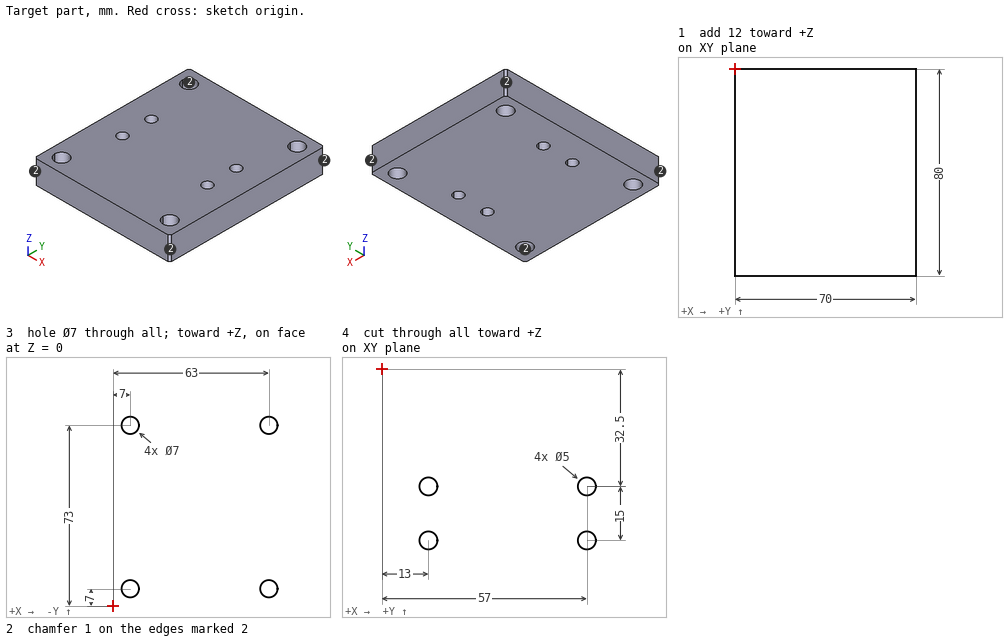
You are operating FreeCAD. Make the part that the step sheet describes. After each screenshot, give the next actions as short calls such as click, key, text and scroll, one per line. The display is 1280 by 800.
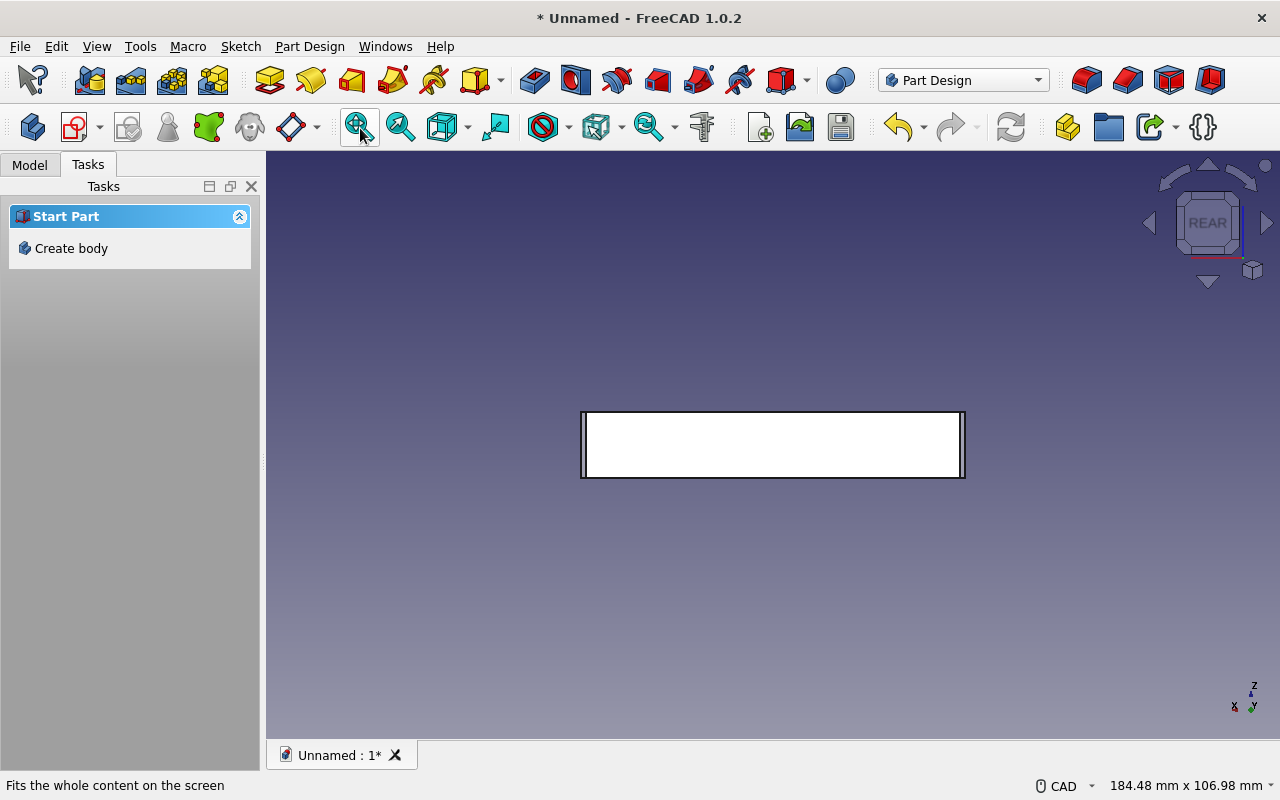
key(5)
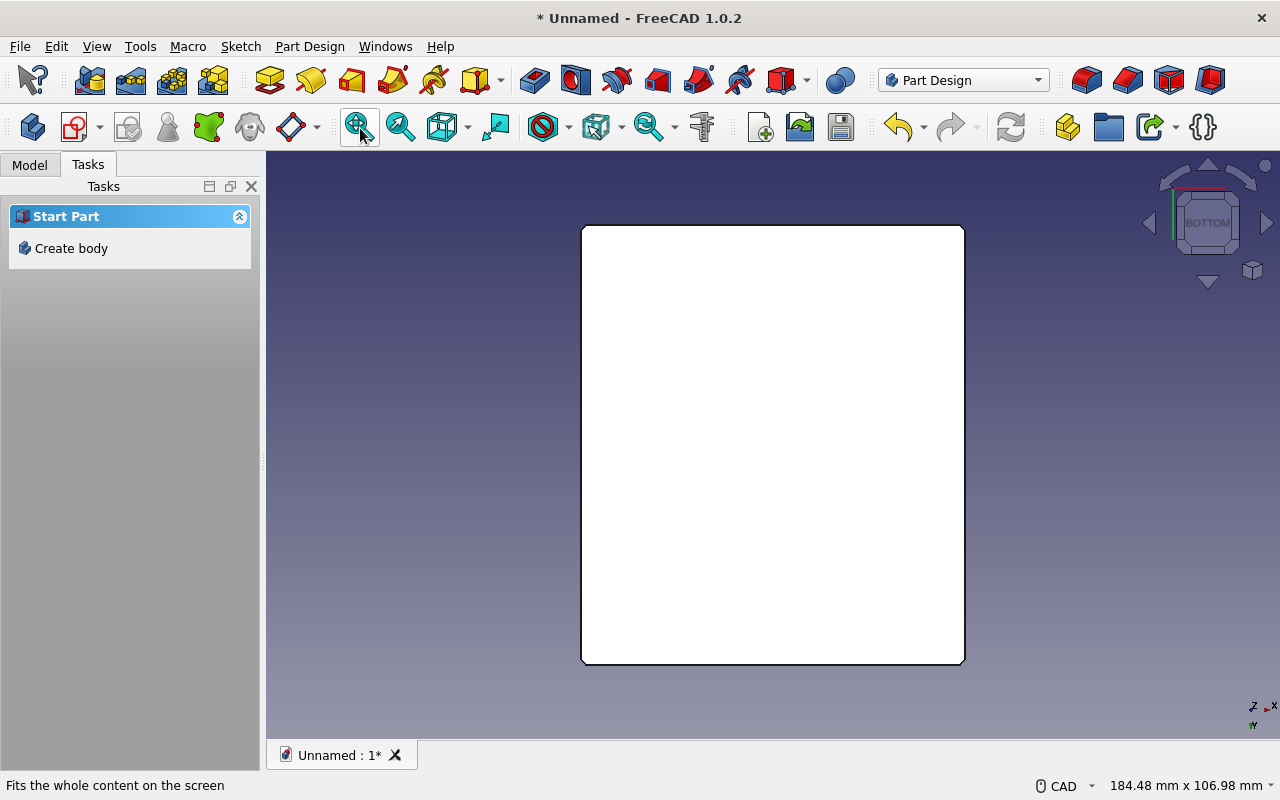
click(773, 444)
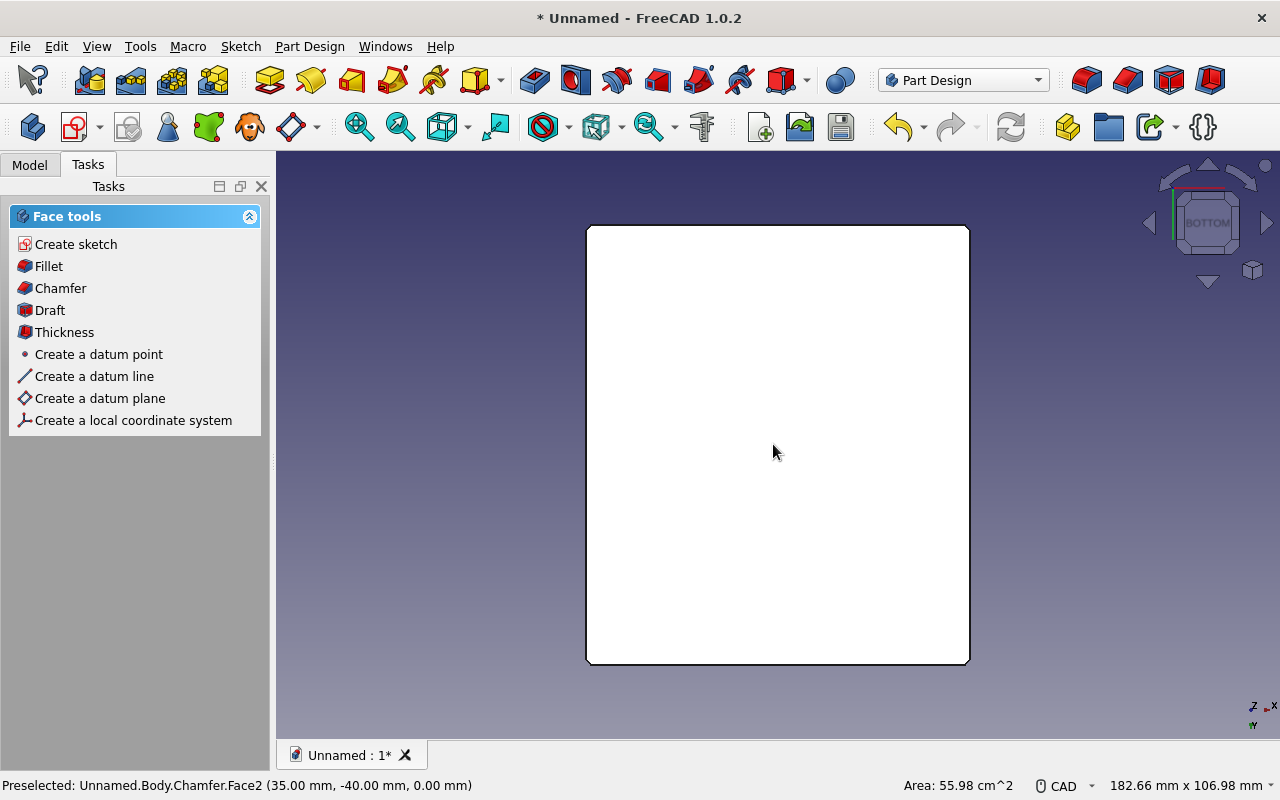
click(74, 128)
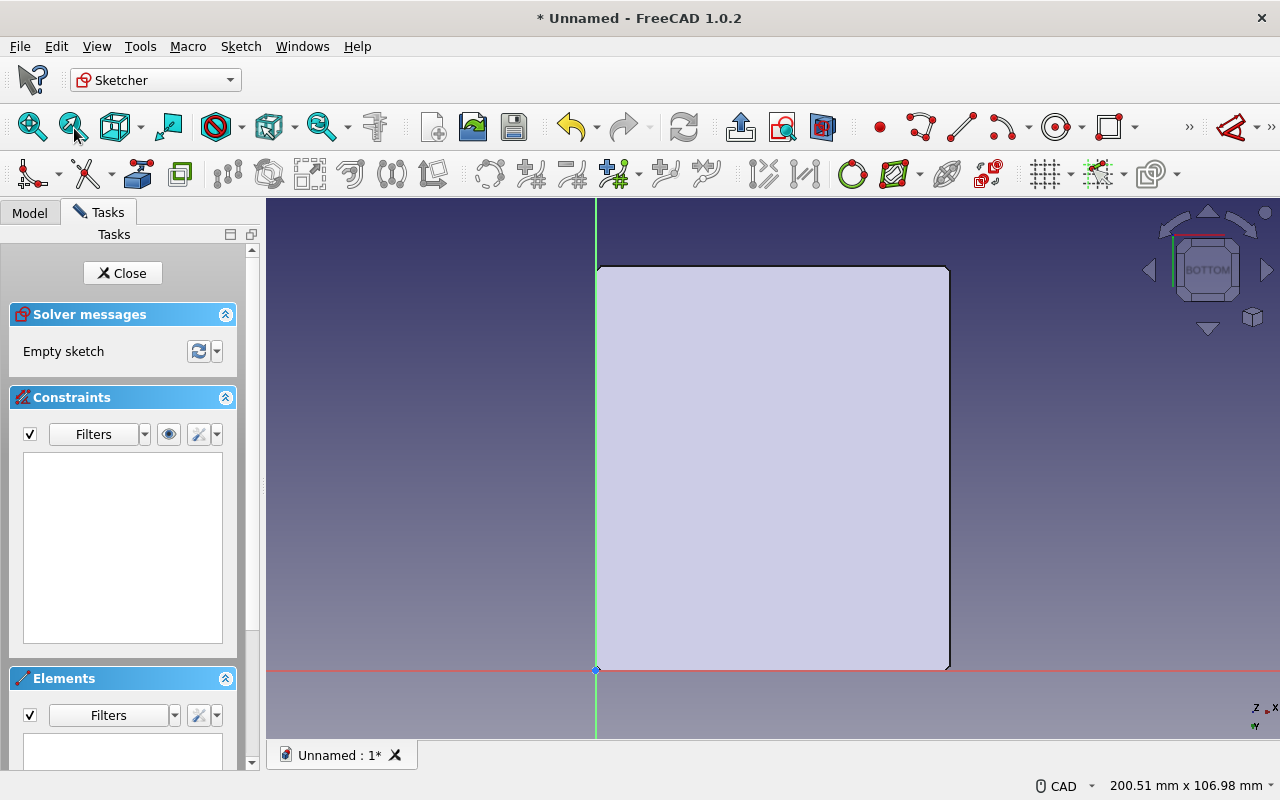
click(1056, 128)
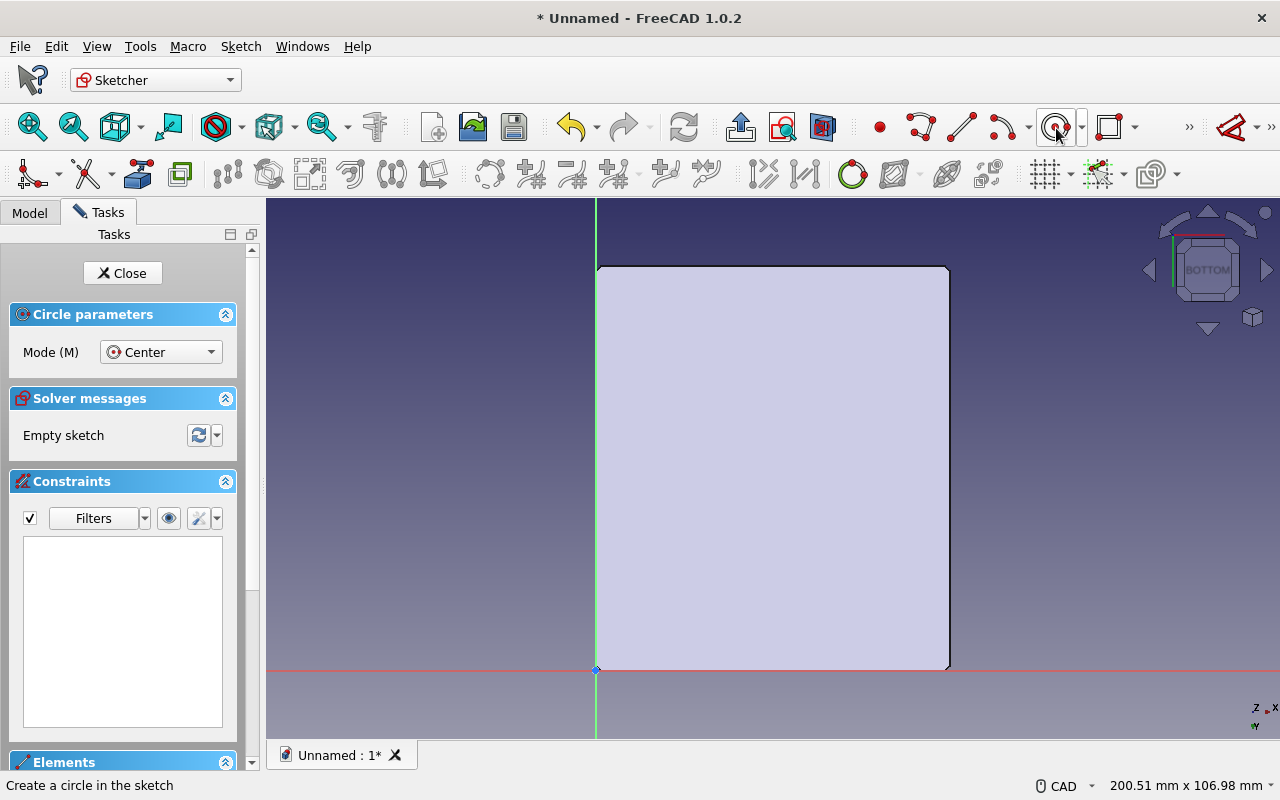
scroll(631, 302, up, 2)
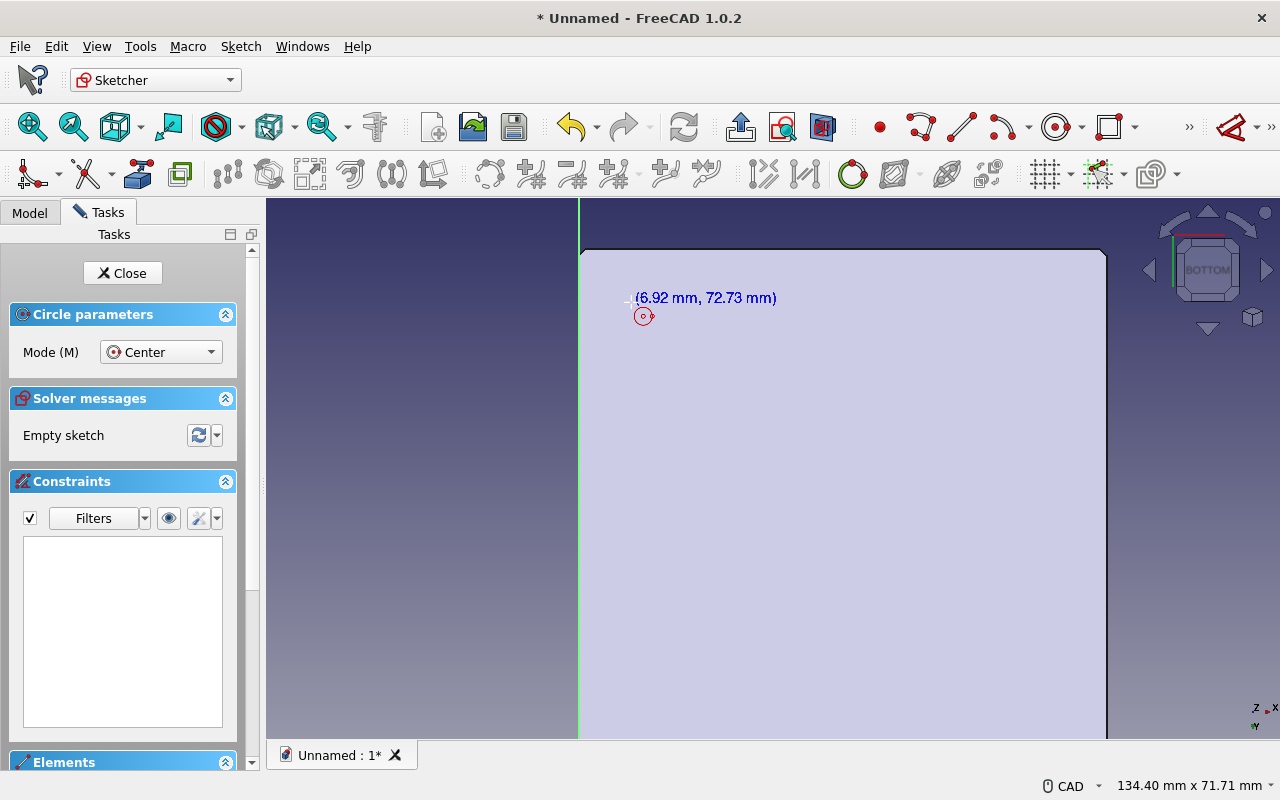
click(631, 301)
move(650, 283)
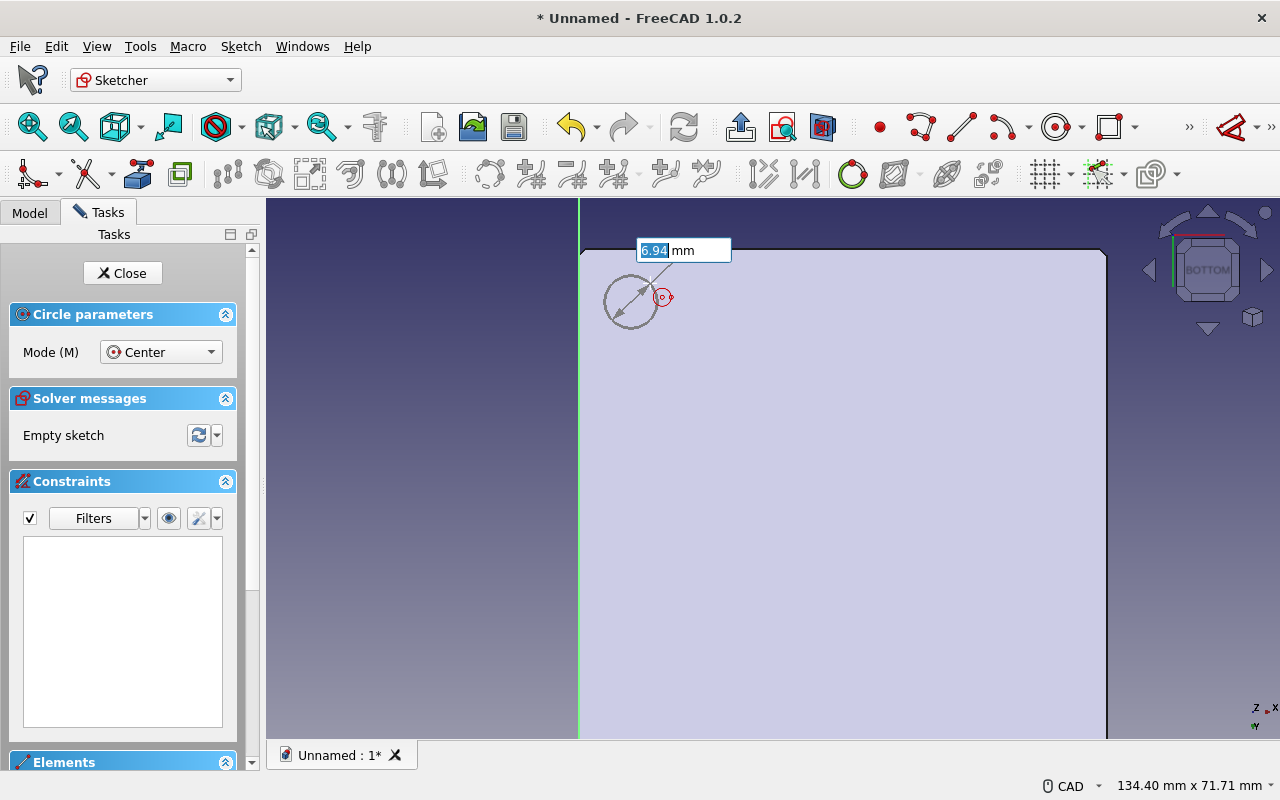
text(7)
key(Return)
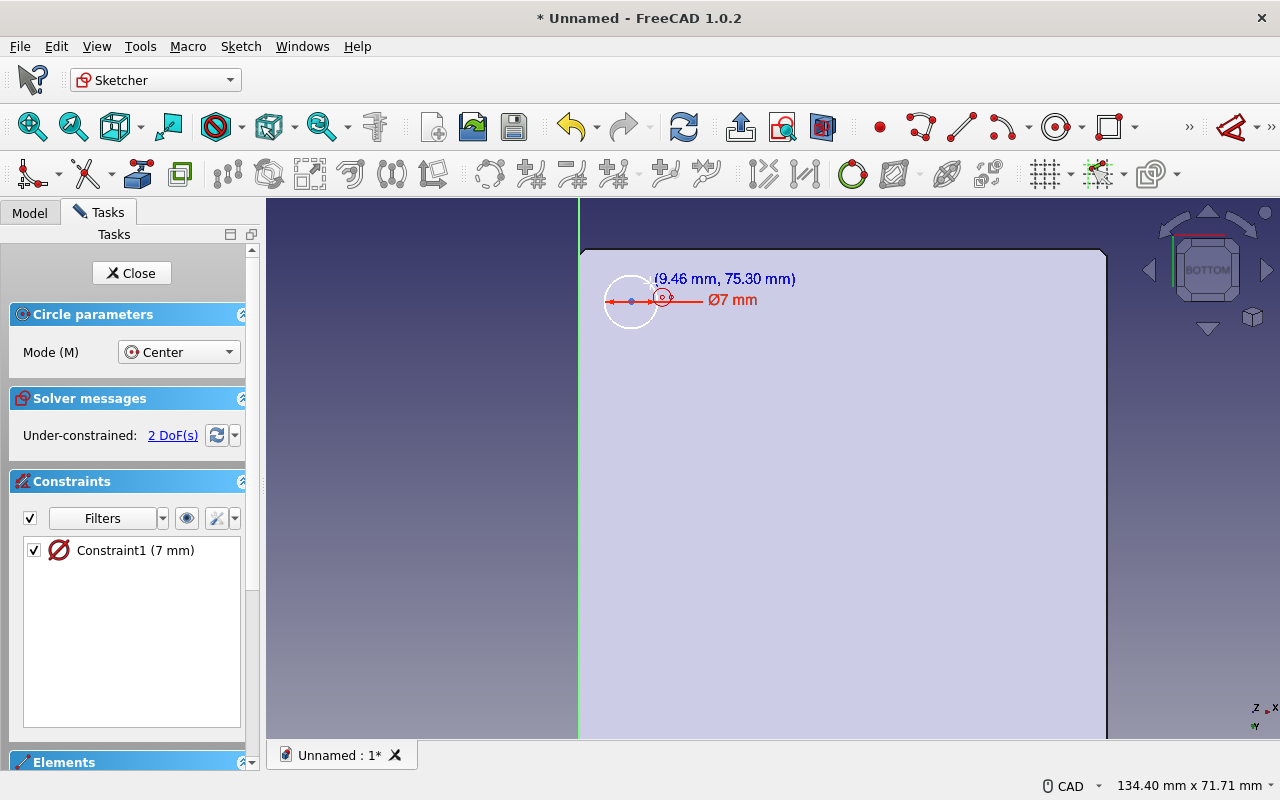
scroll(553, 353, down, 3)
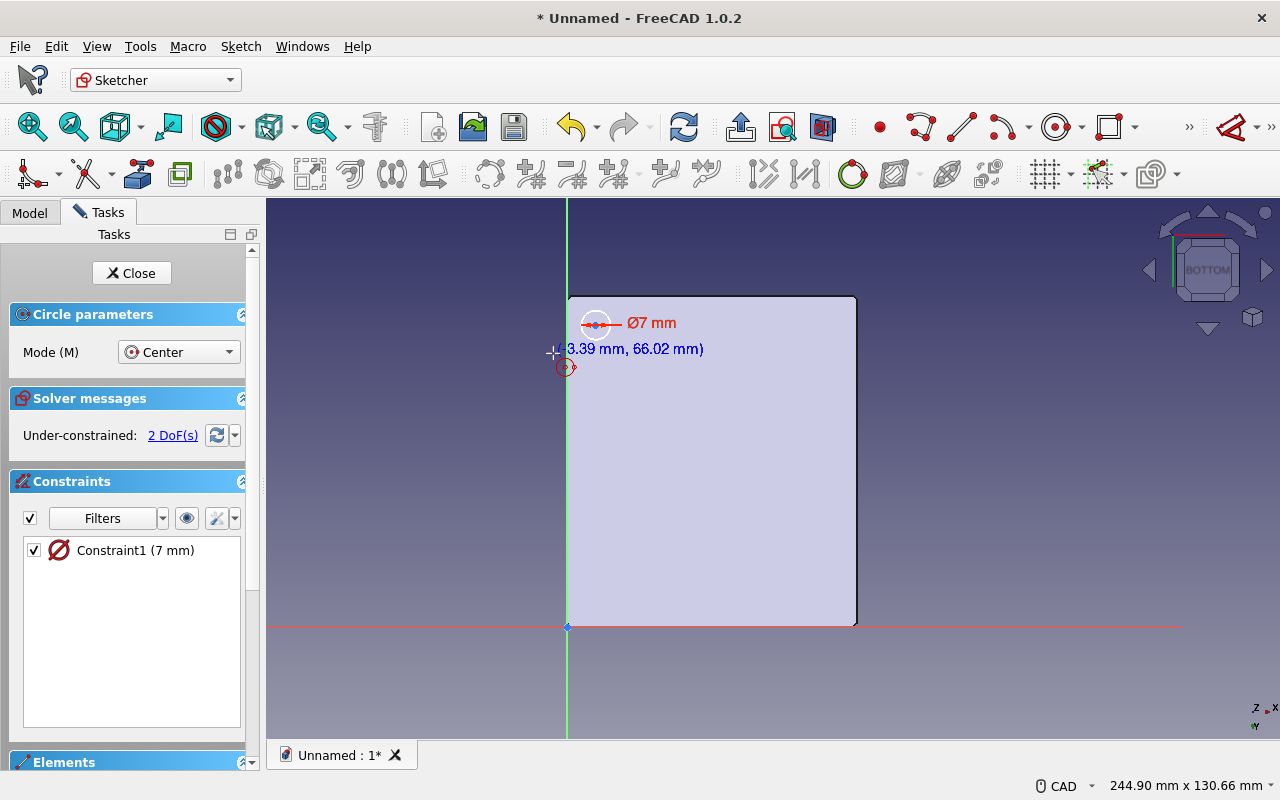
scroll(596, 598, up, 3)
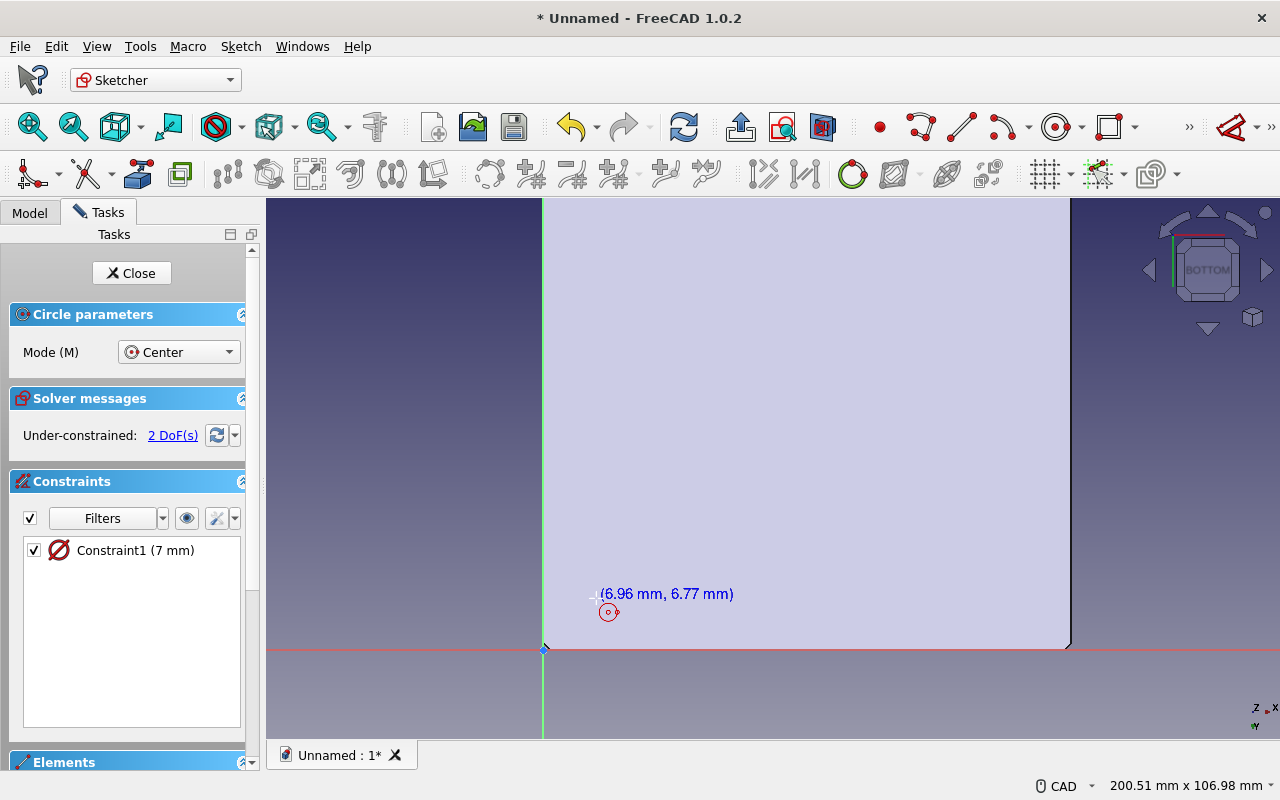
click(596, 597)
move(615, 579)